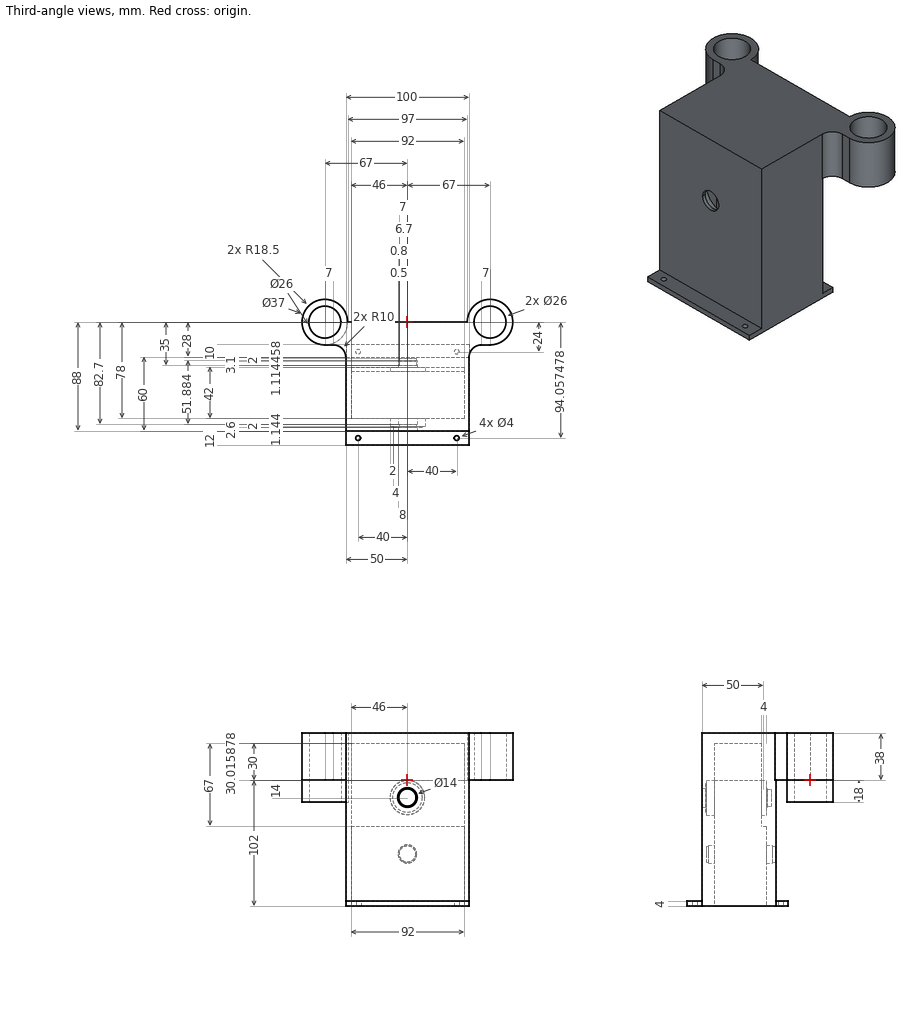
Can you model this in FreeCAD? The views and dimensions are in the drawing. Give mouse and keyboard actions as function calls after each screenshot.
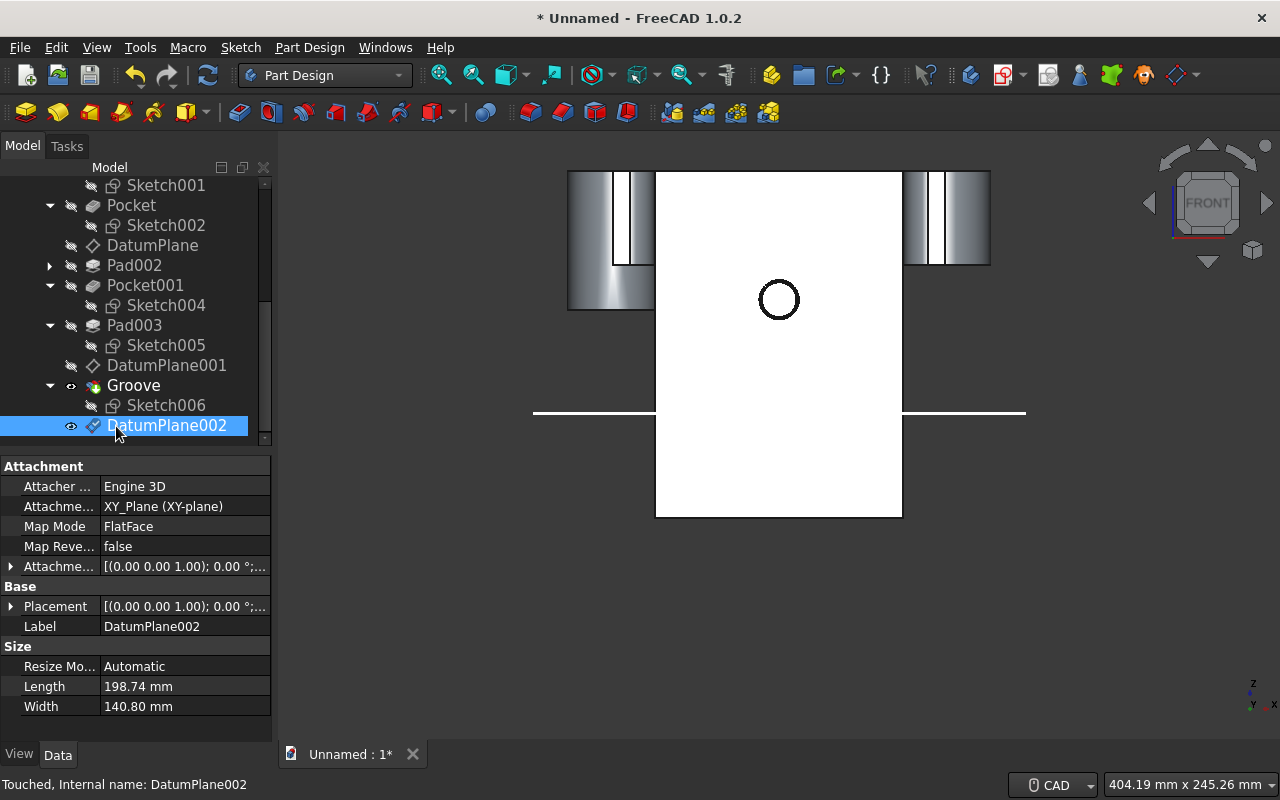
click(1004, 76)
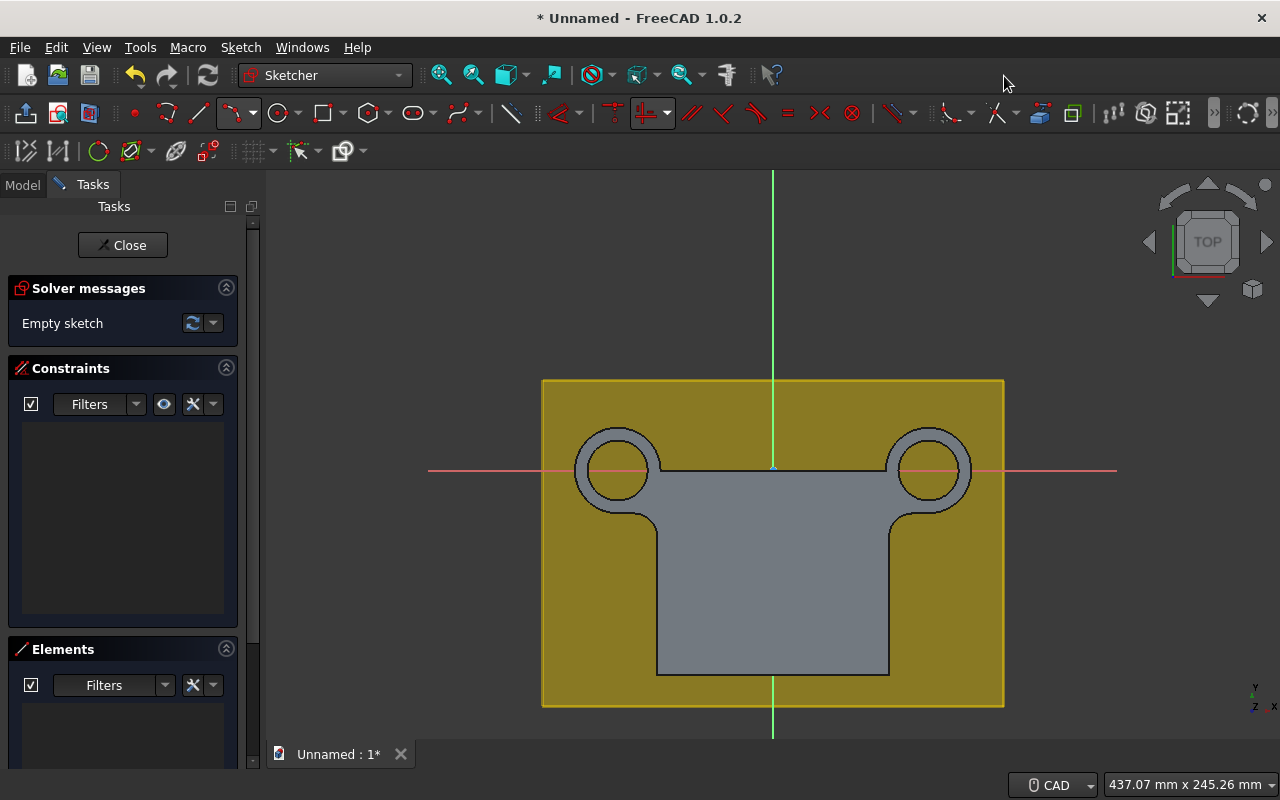
key(q)
key(s)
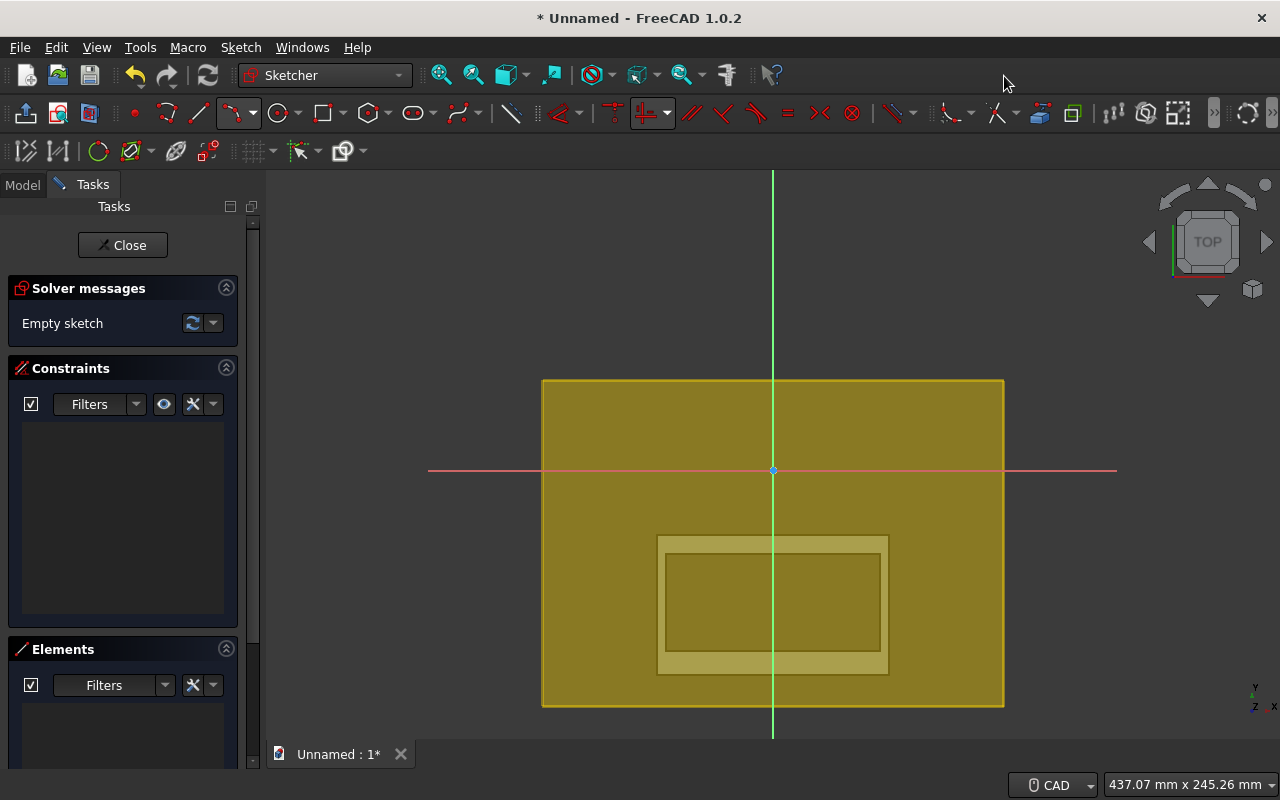
scroll(837, 708, up, 3)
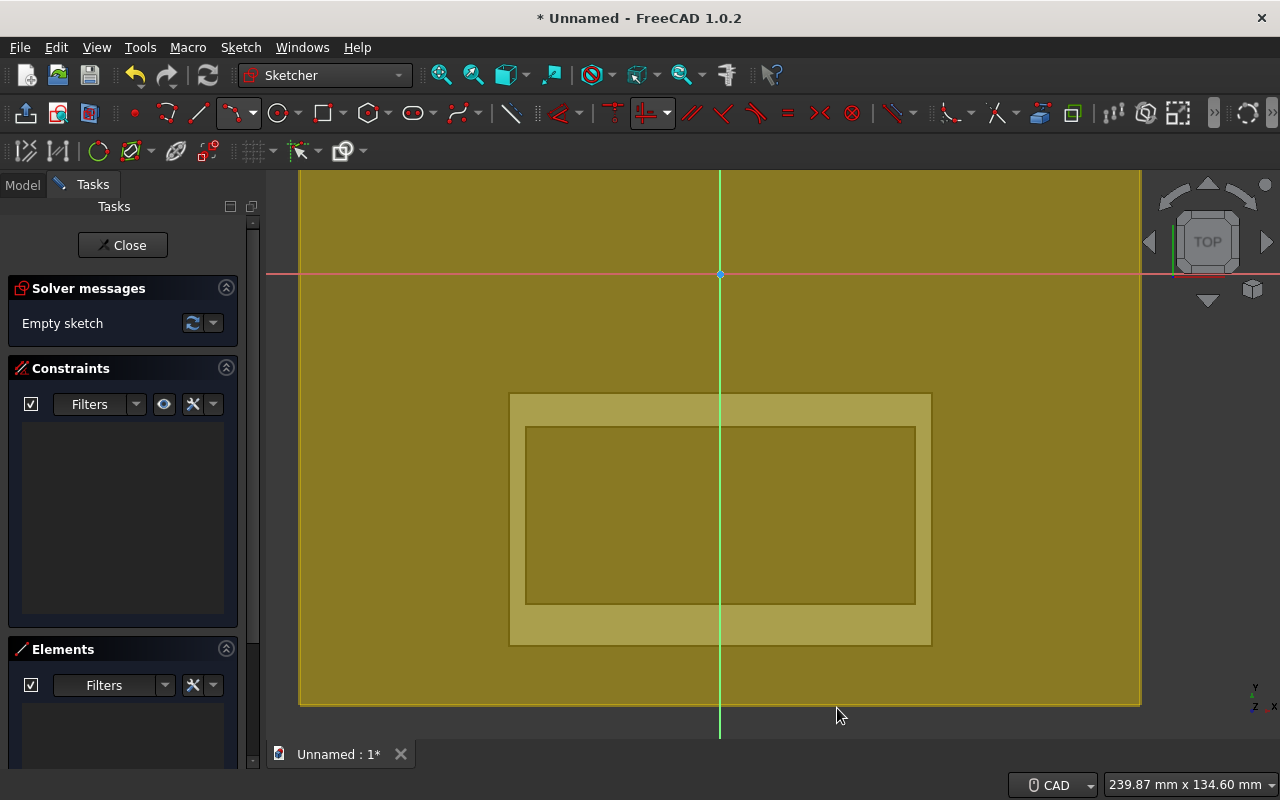
key(g)
key(m)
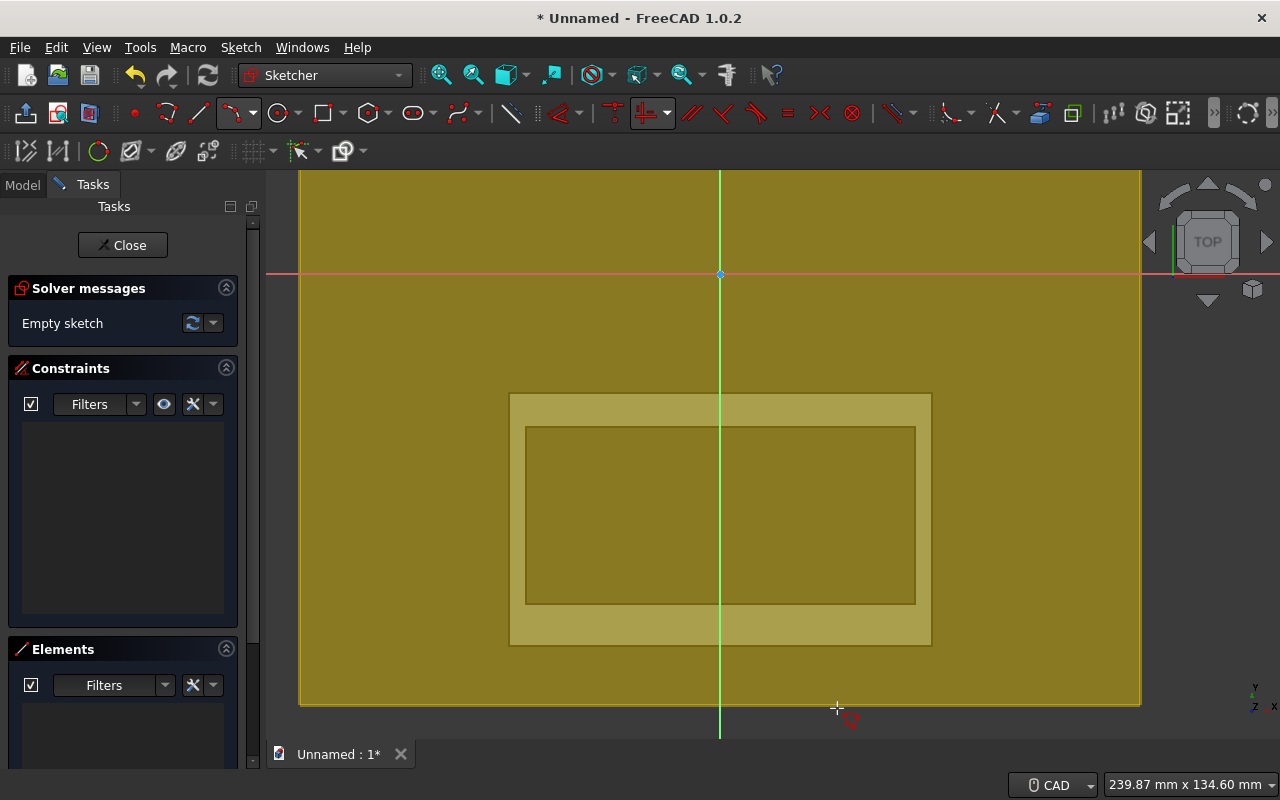
click(720, 396)
click(692, 396)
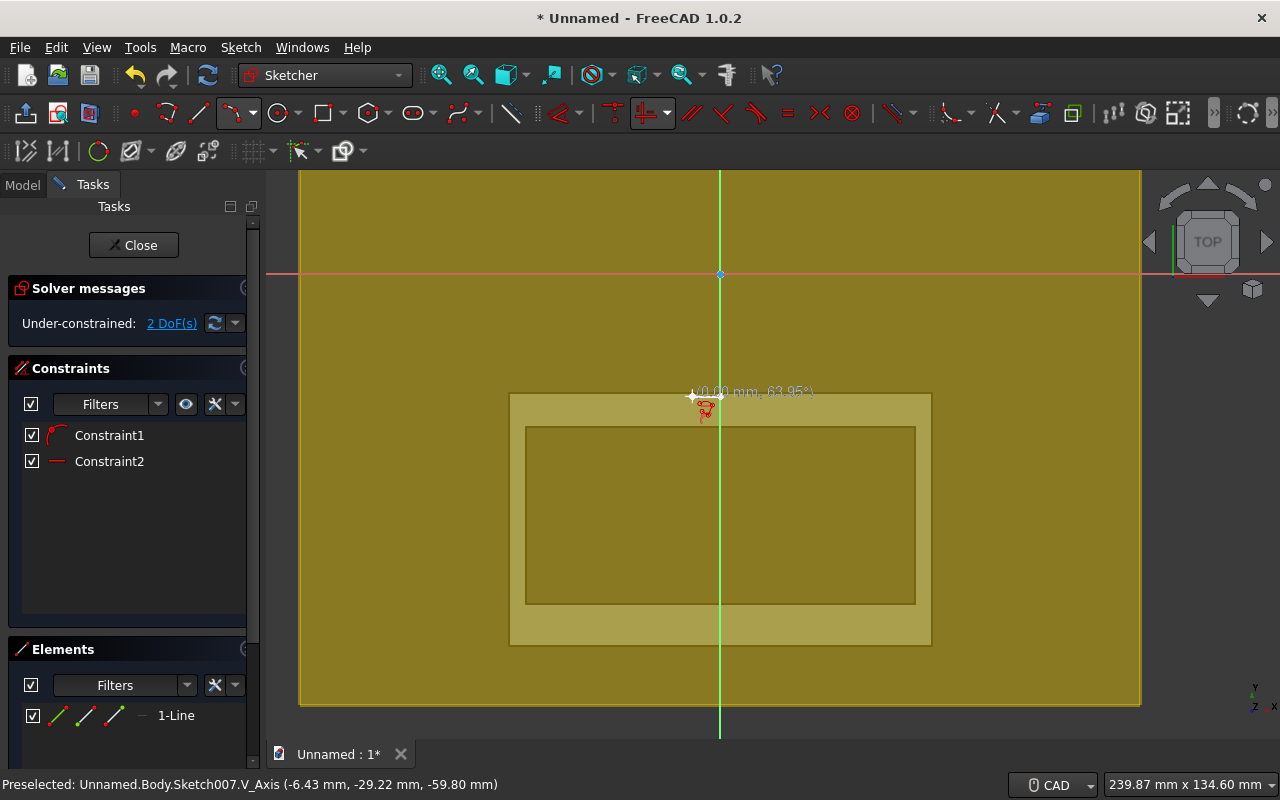
scroll(692, 405, up, 4)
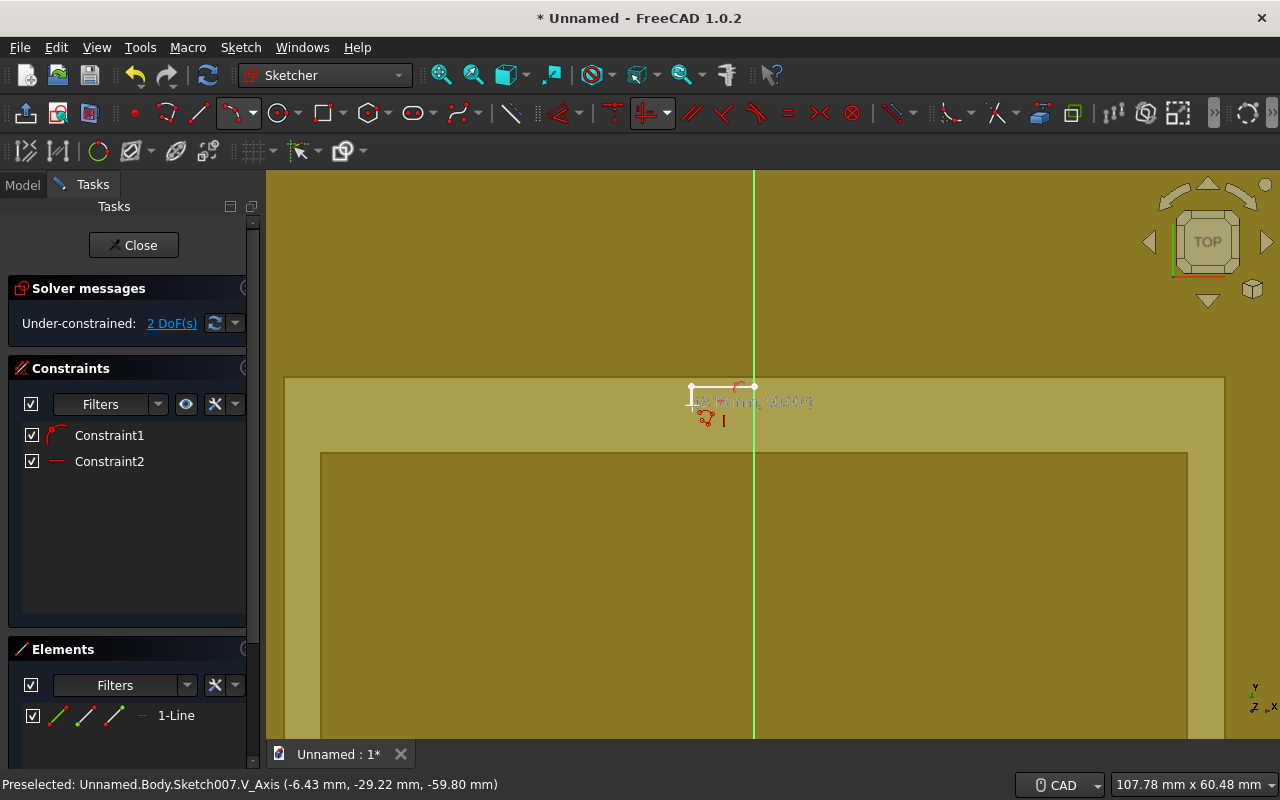
click(691, 404)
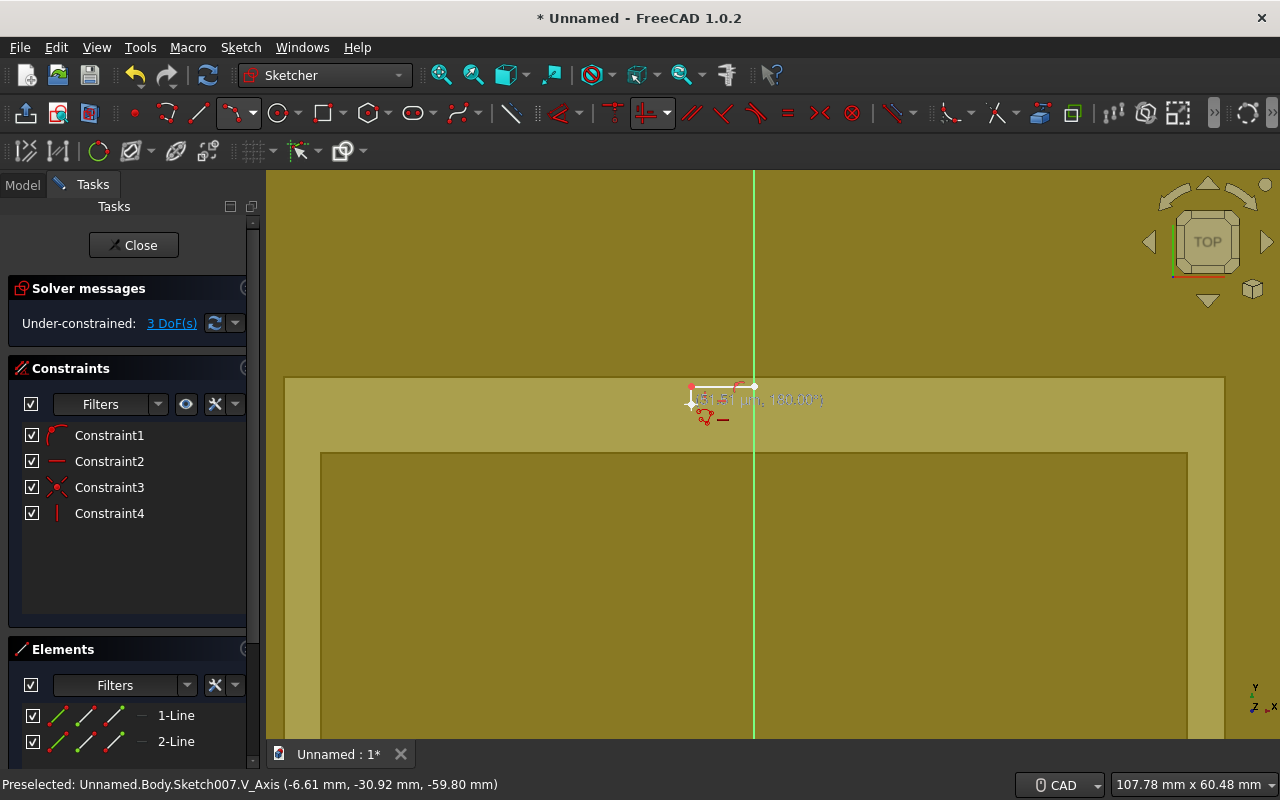
scroll(684, 404, up, 4)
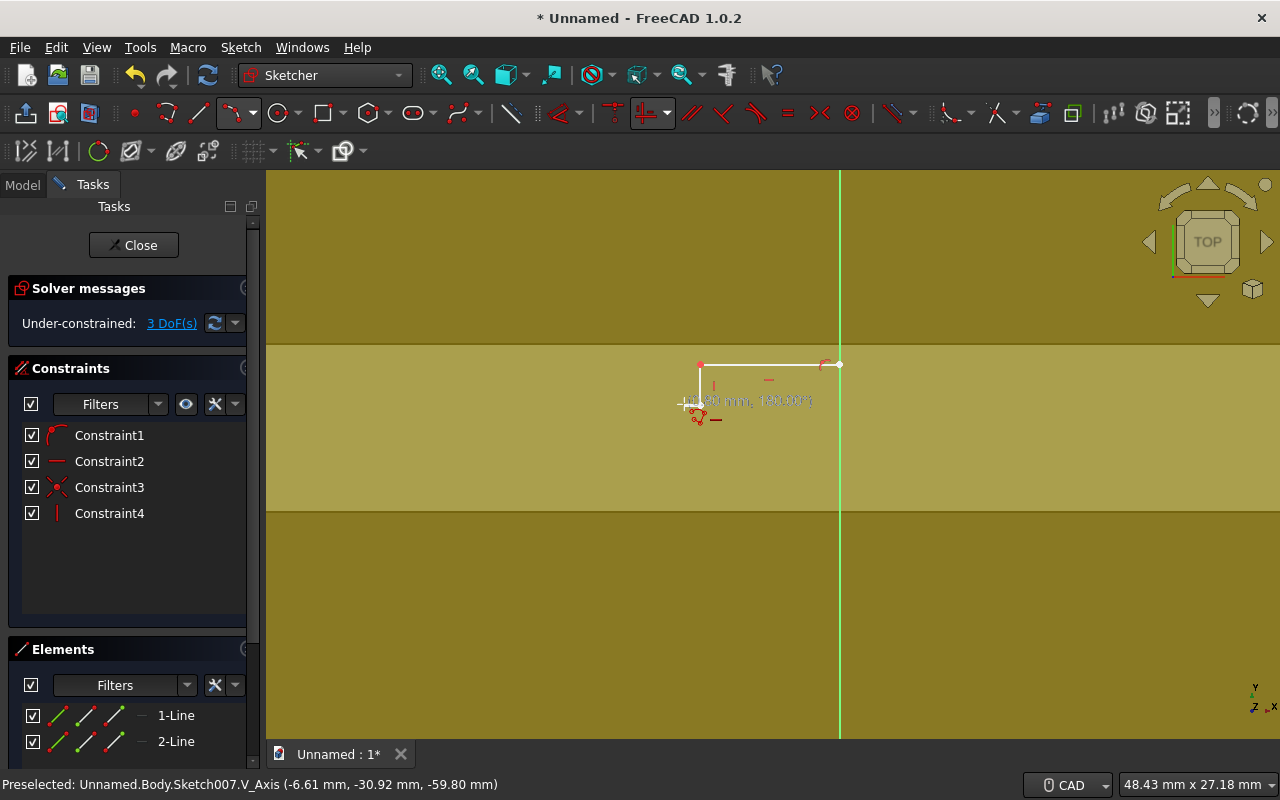
click(683, 403)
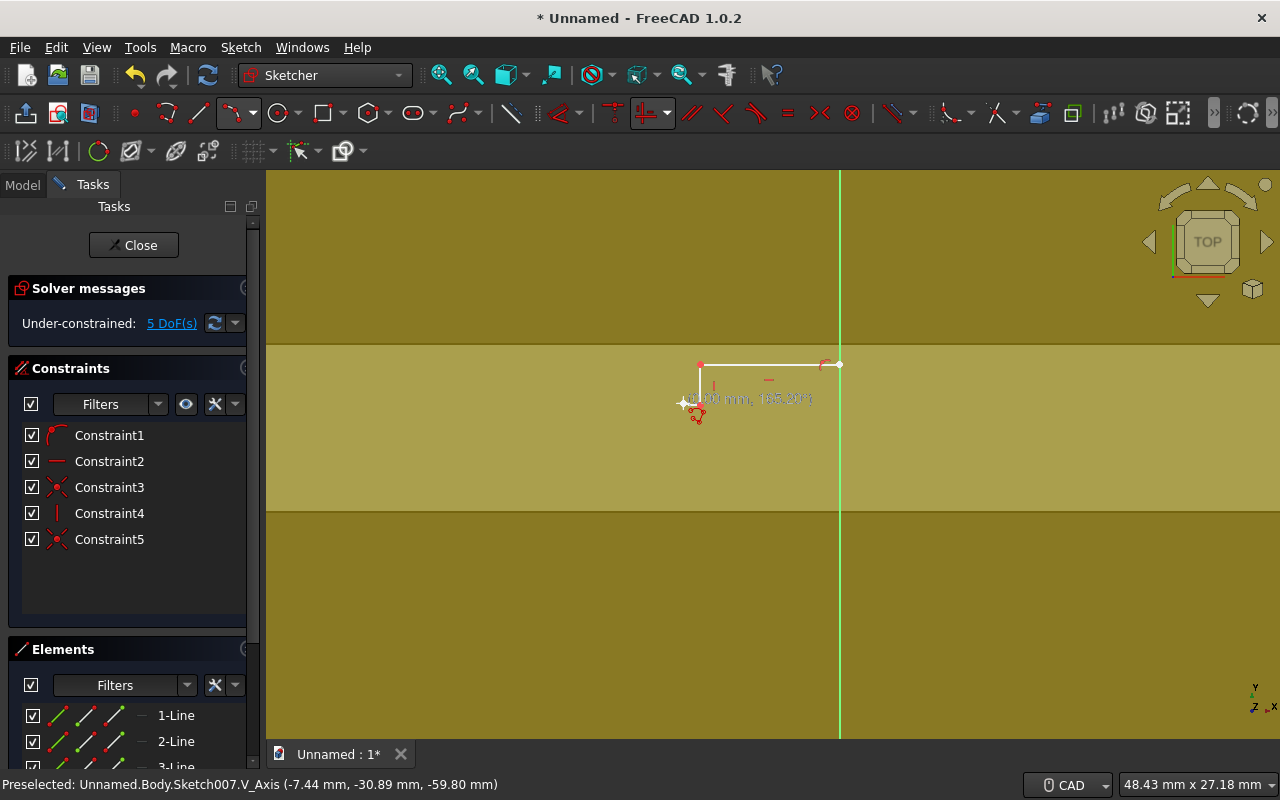
scroll(690, 406, down, 8)